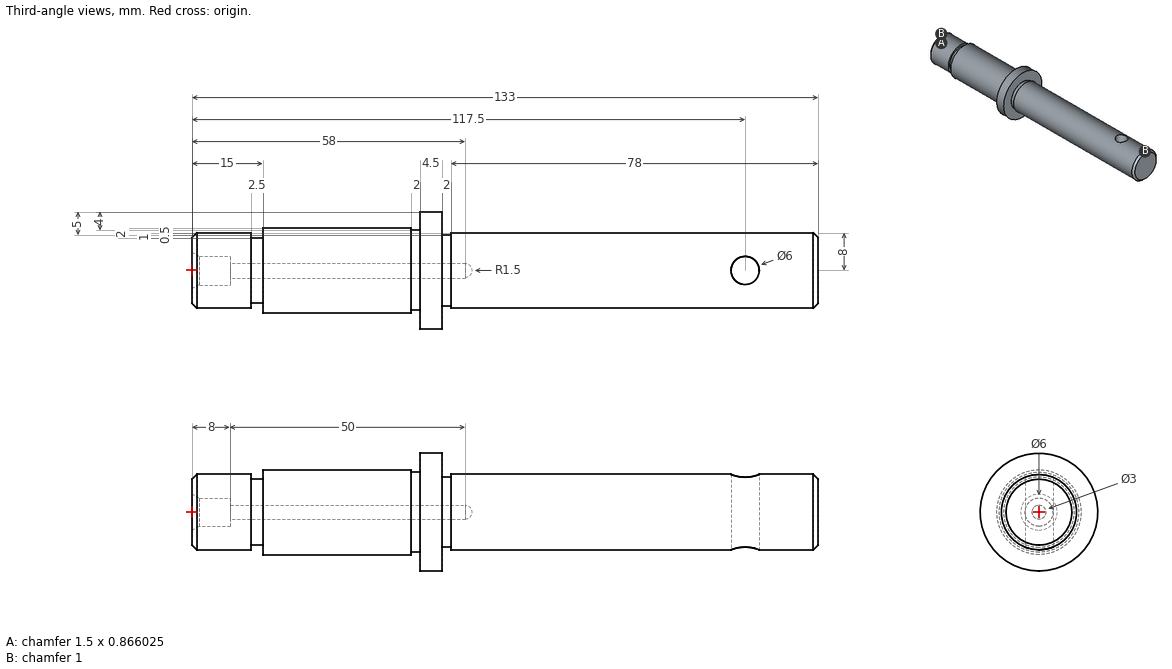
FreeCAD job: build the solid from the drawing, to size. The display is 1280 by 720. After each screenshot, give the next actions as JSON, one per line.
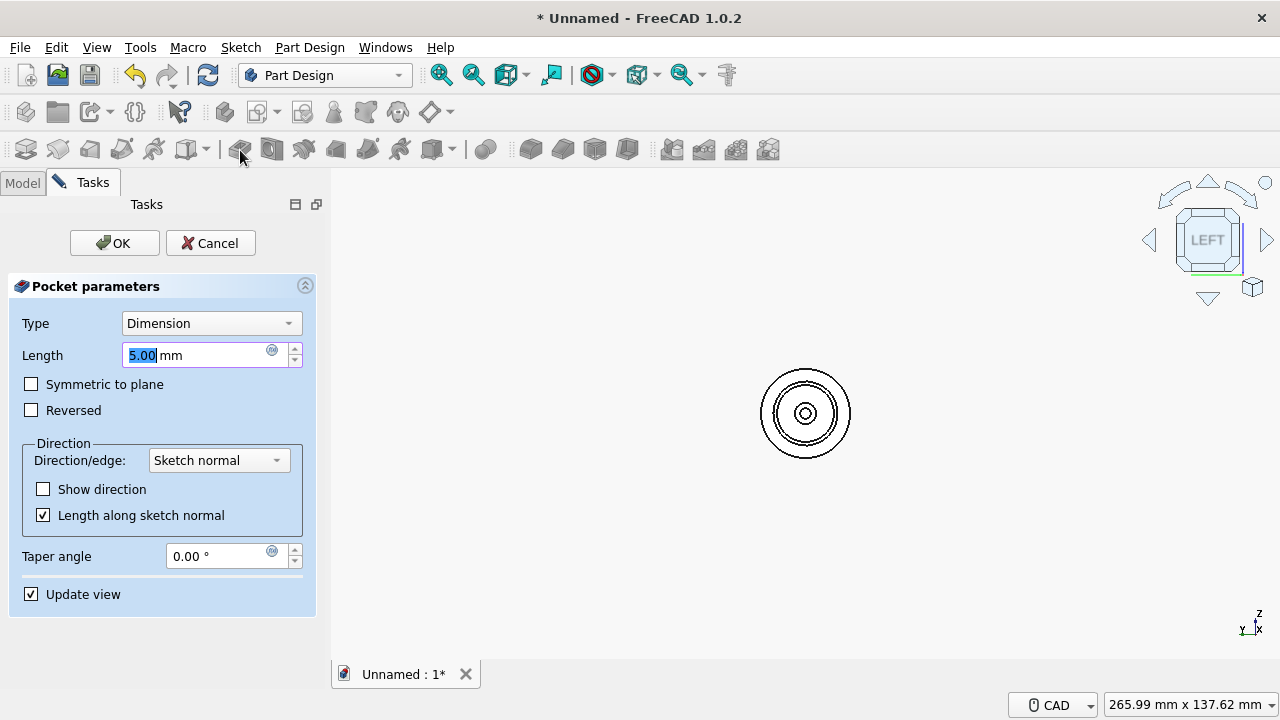
{"action": "type", "text": "50"}
{"action": "key", "text": "Tab"}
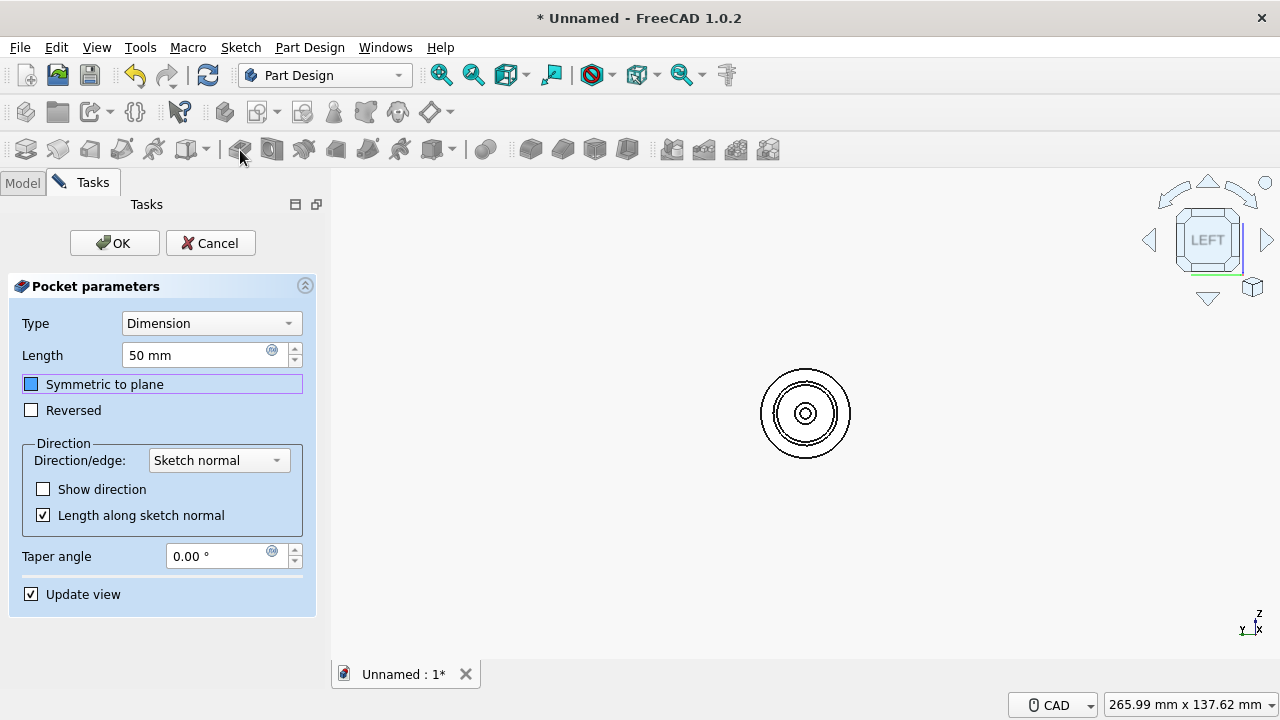
{"action": "left_click", "coordinate": [115, 243]}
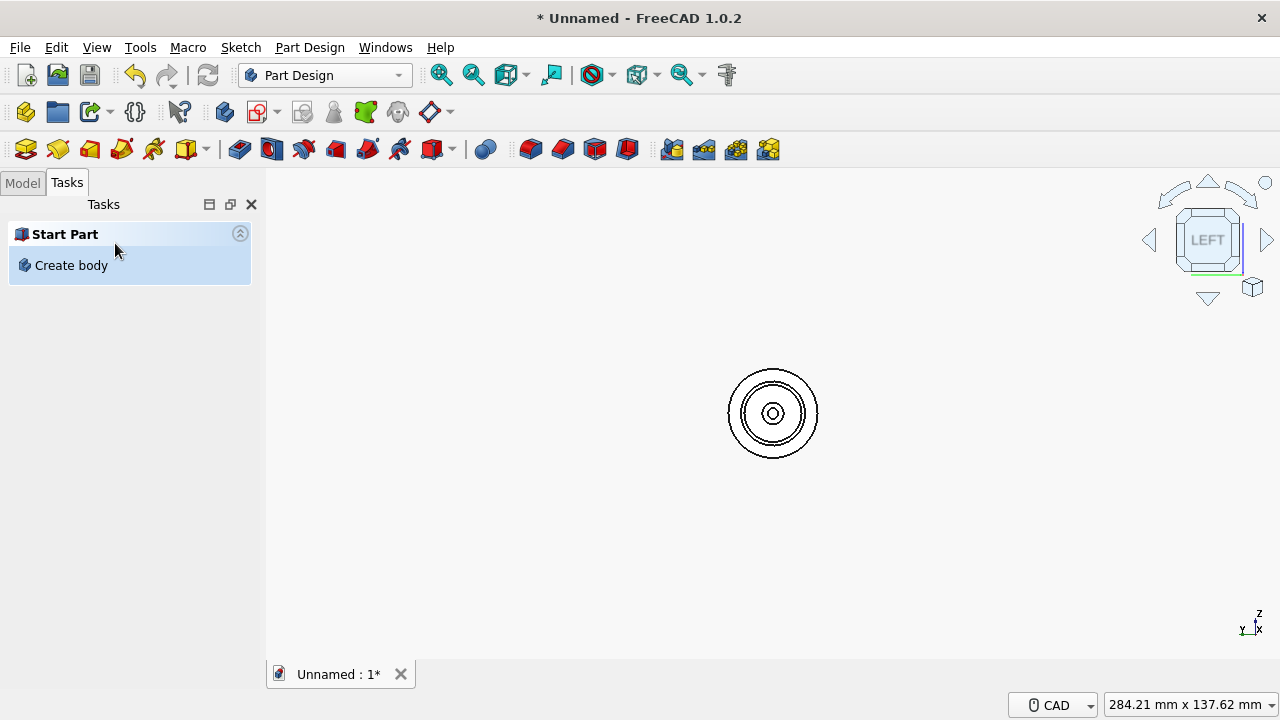
{"action": "left_click", "coordinate": [442, 76]}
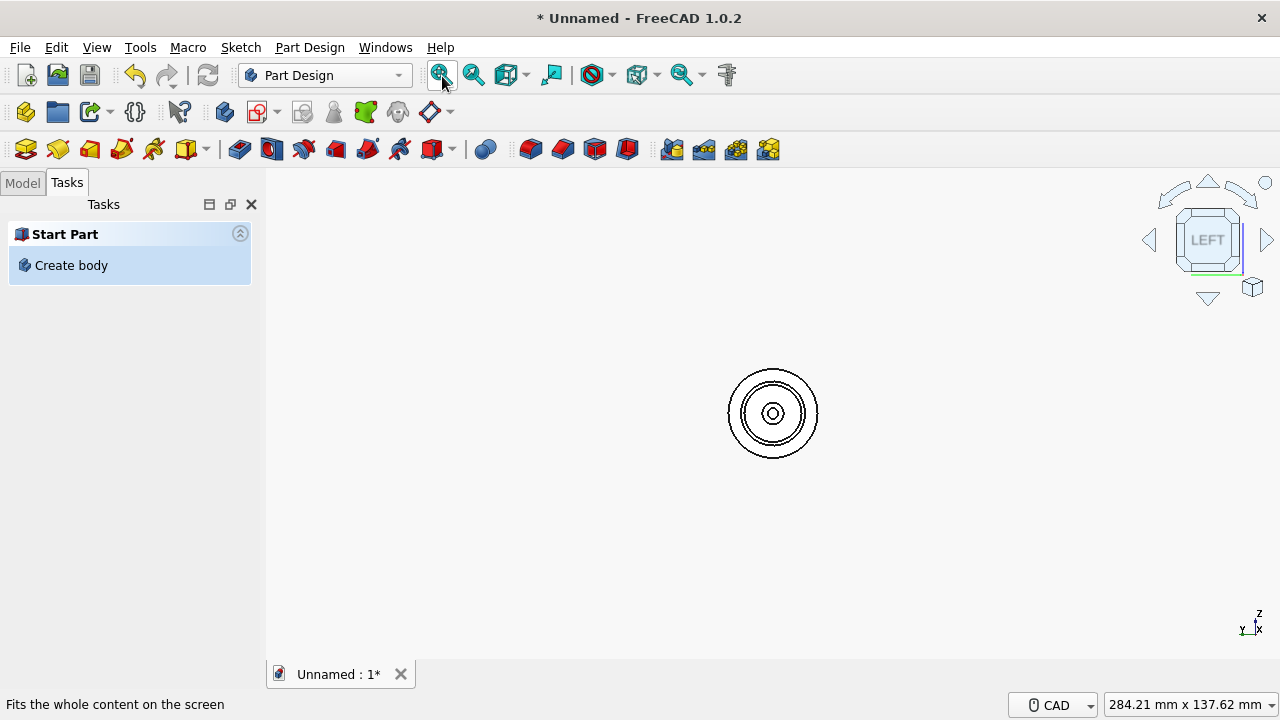
{"action": "left_click", "coordinate": [764, 406]}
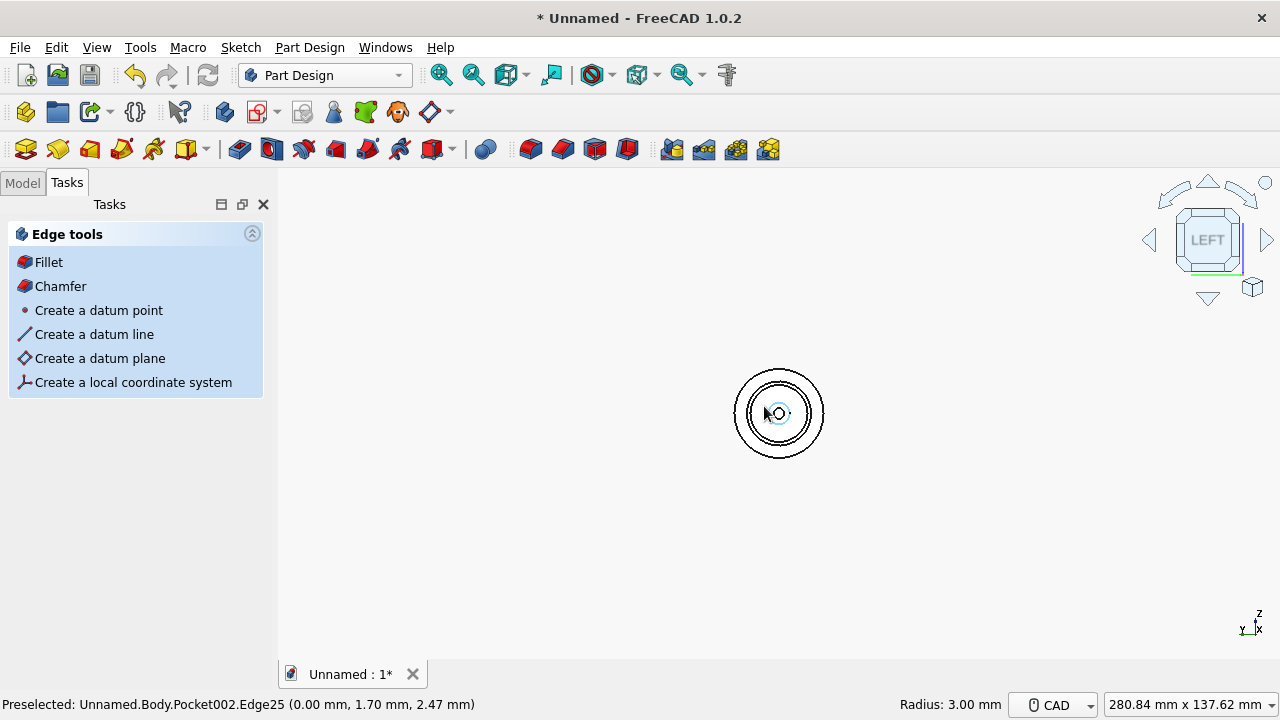
{"action": "left_click", "coordinate": [564, 150]}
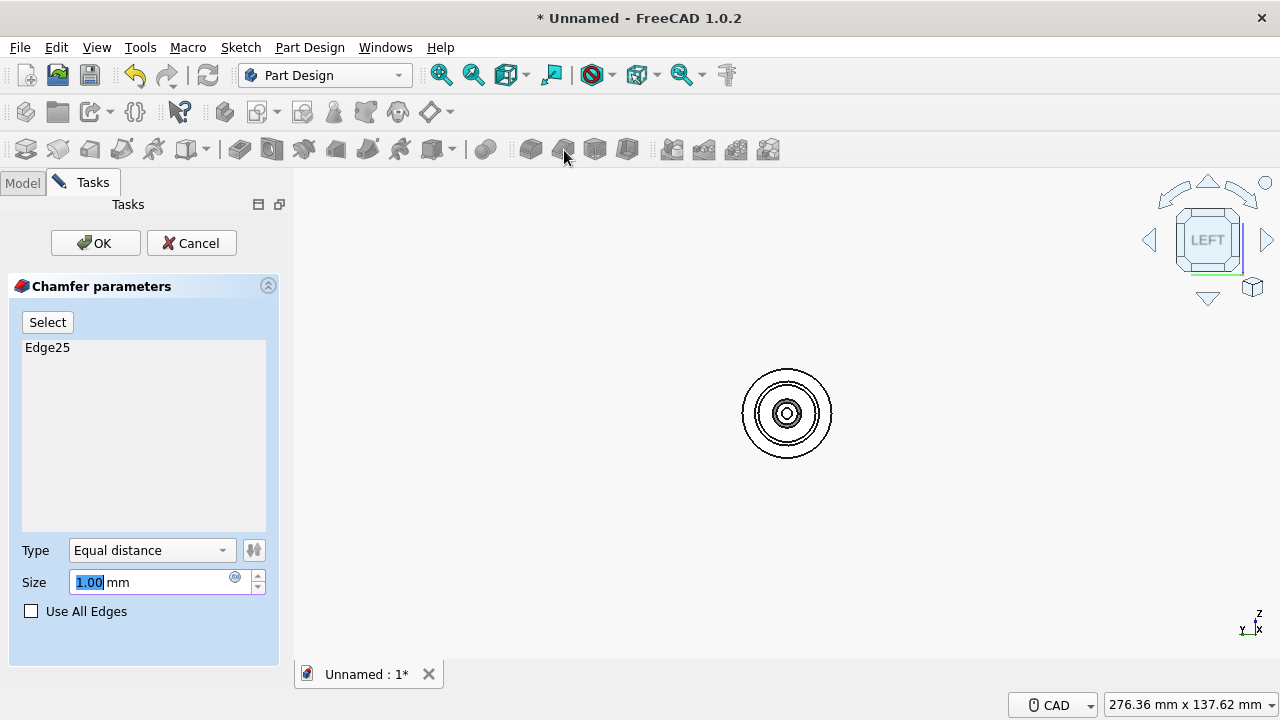
{"action": "type", "text": "1.5"}
{"action": "key", "text": "Tab"}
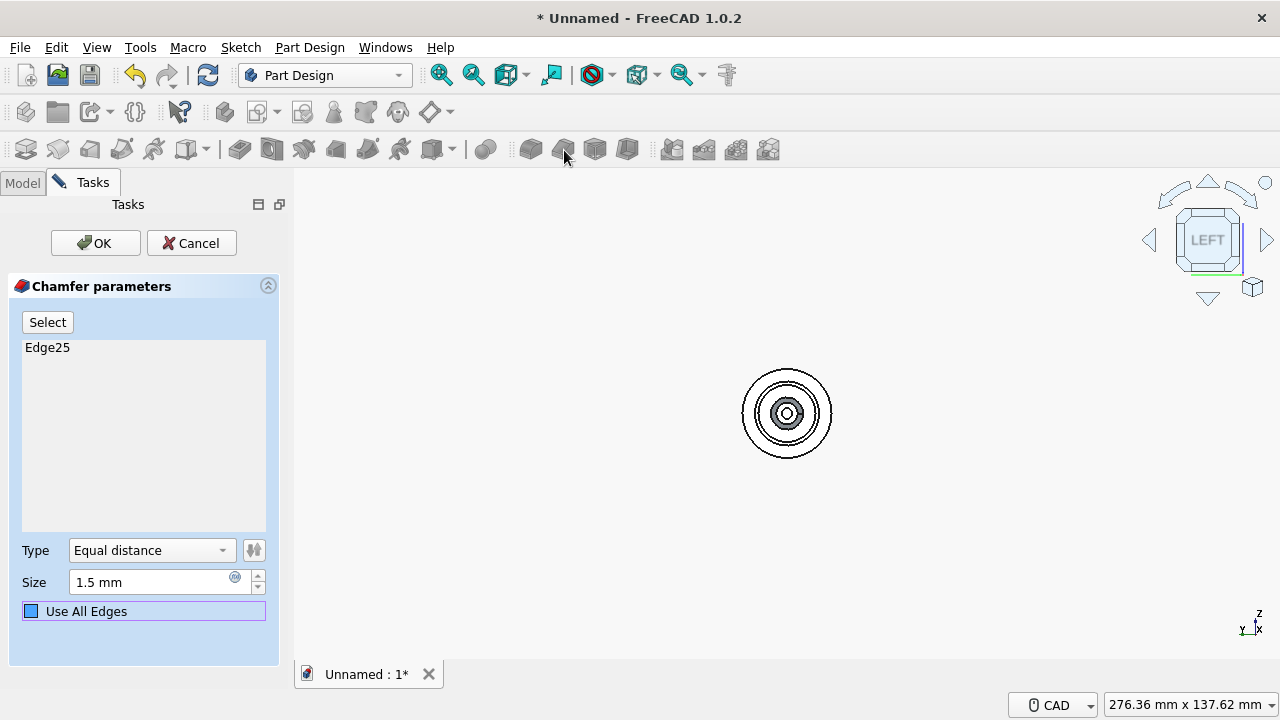
{"action": "left_click", "coordinate": [153, 550]}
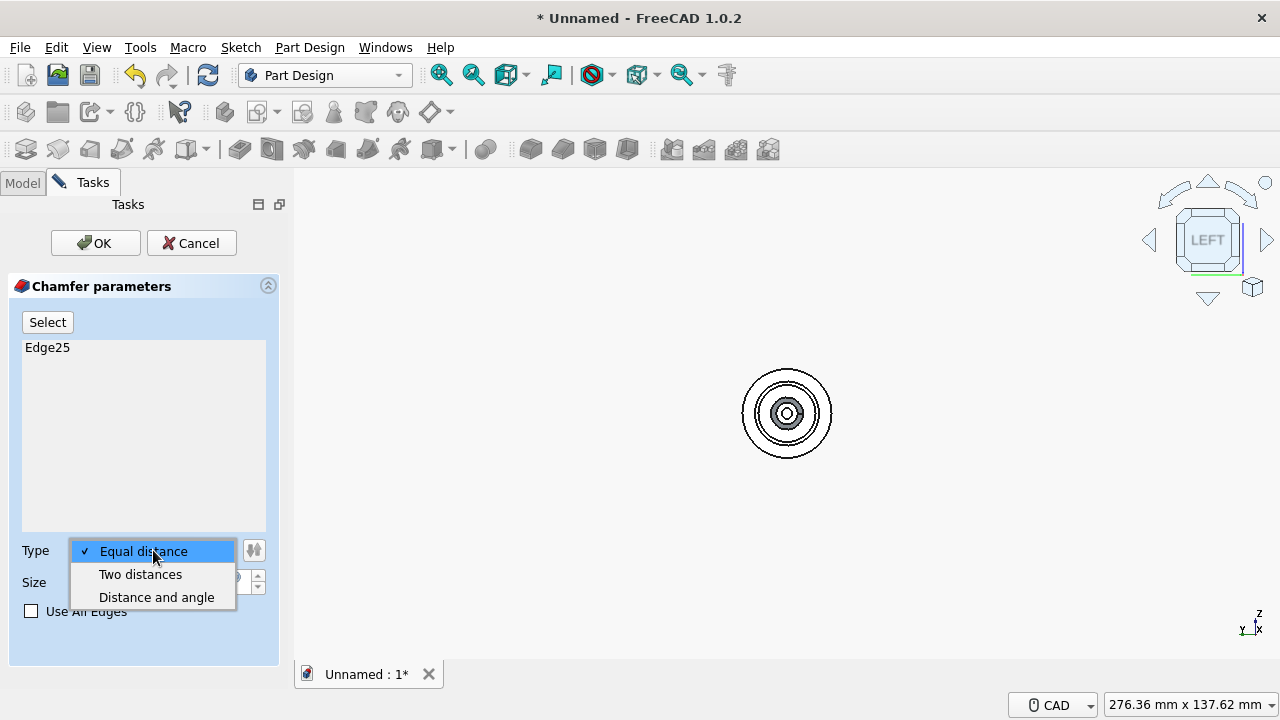
{"action": "left_click", "coordinate": [152, 574]}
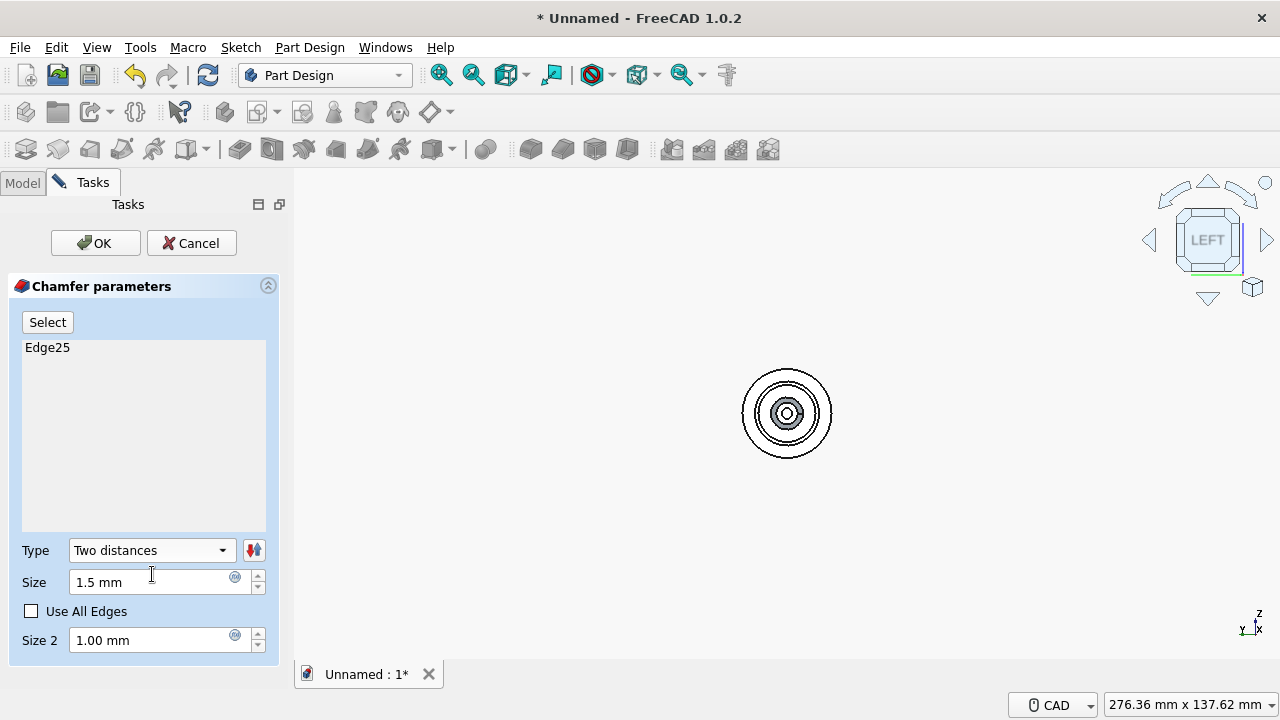
{"action": "triple_click", "coordinate": [160, 640]}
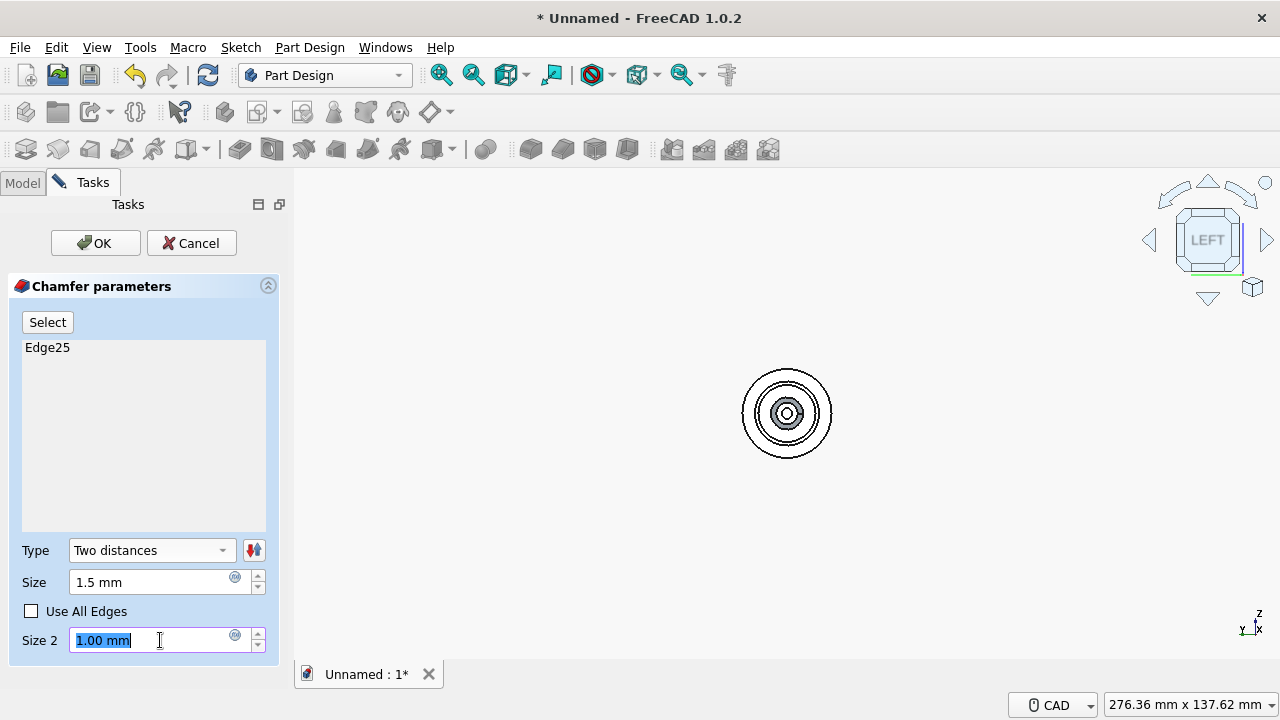
{"action": "type", "text": "0.866025"}
{"action": "key", "text": "Tab"}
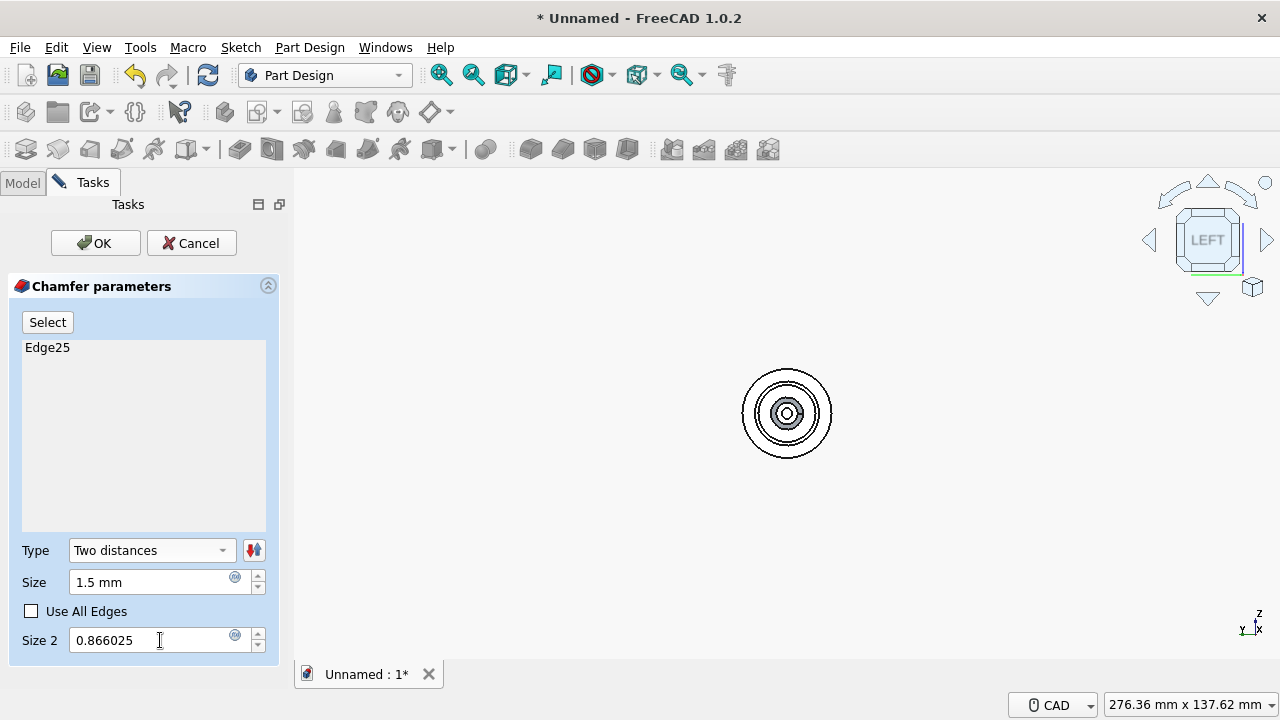
{"action": "left_click", "coordinate": [254, 550]}